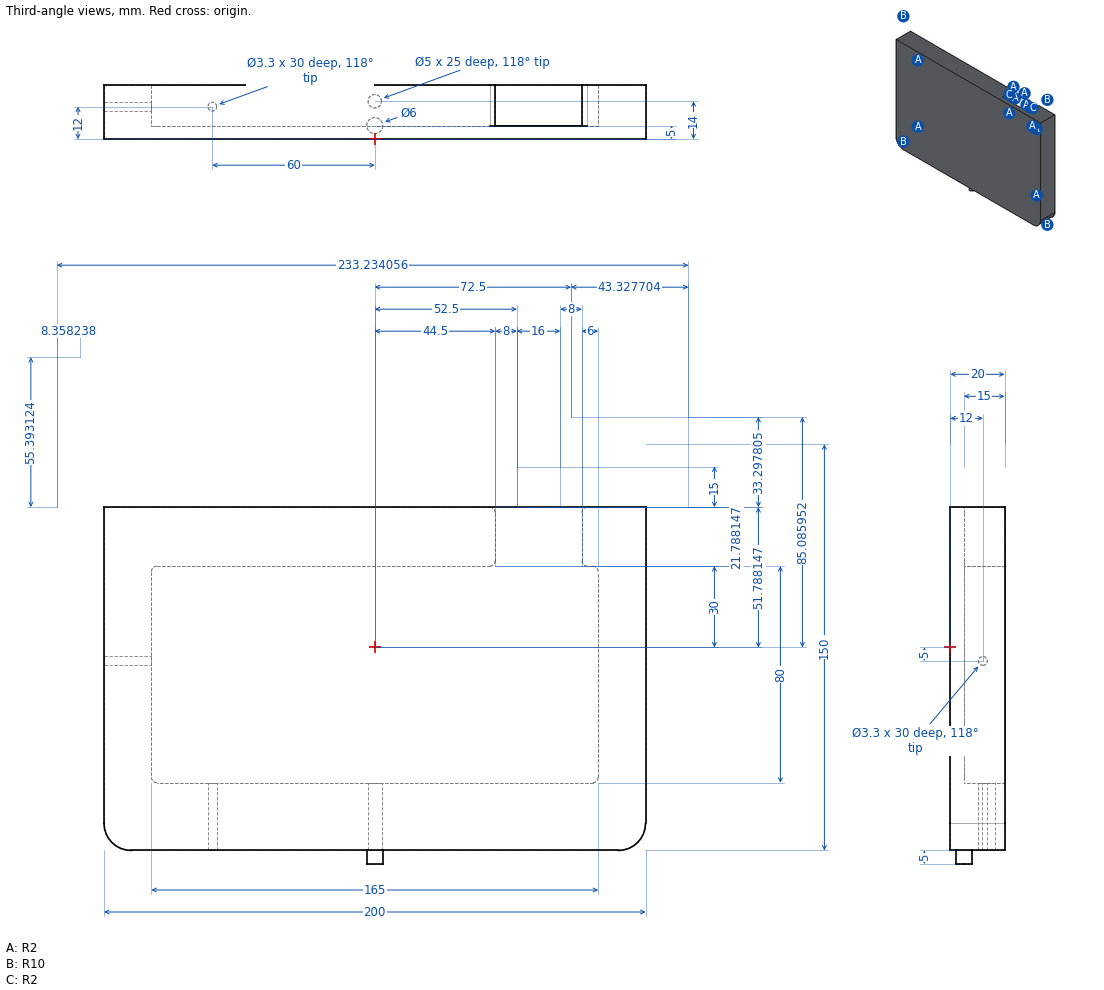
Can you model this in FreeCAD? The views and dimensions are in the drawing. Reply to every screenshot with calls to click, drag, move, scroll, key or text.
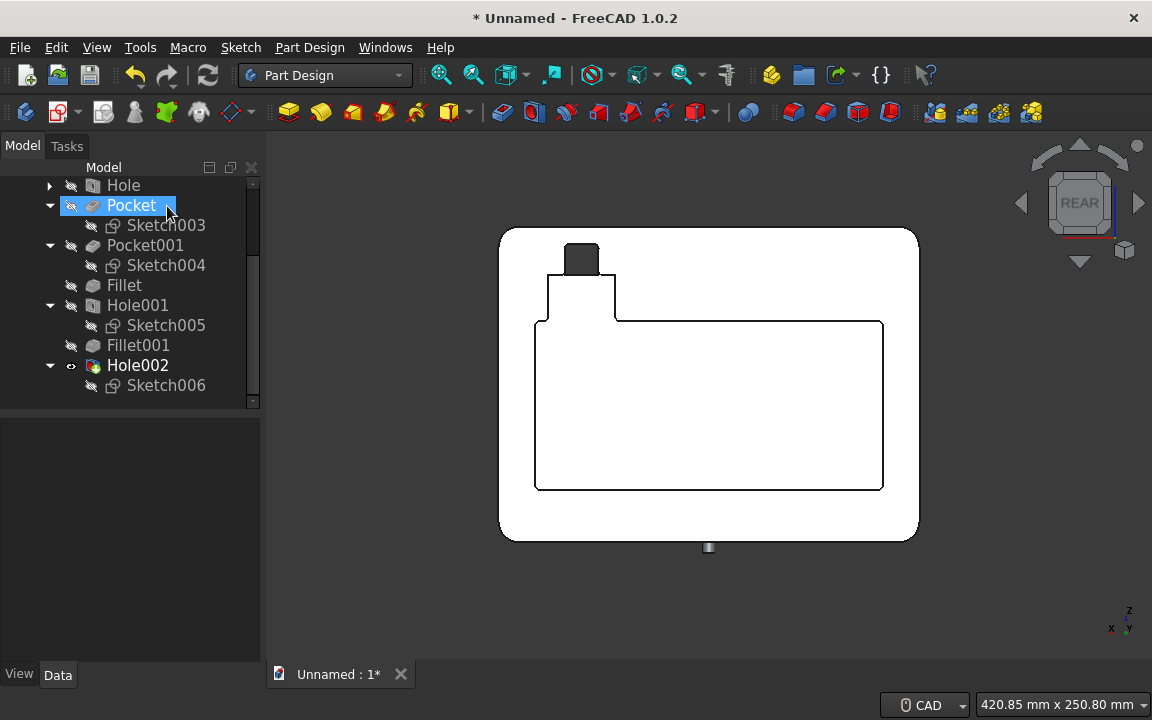
click(889, 293)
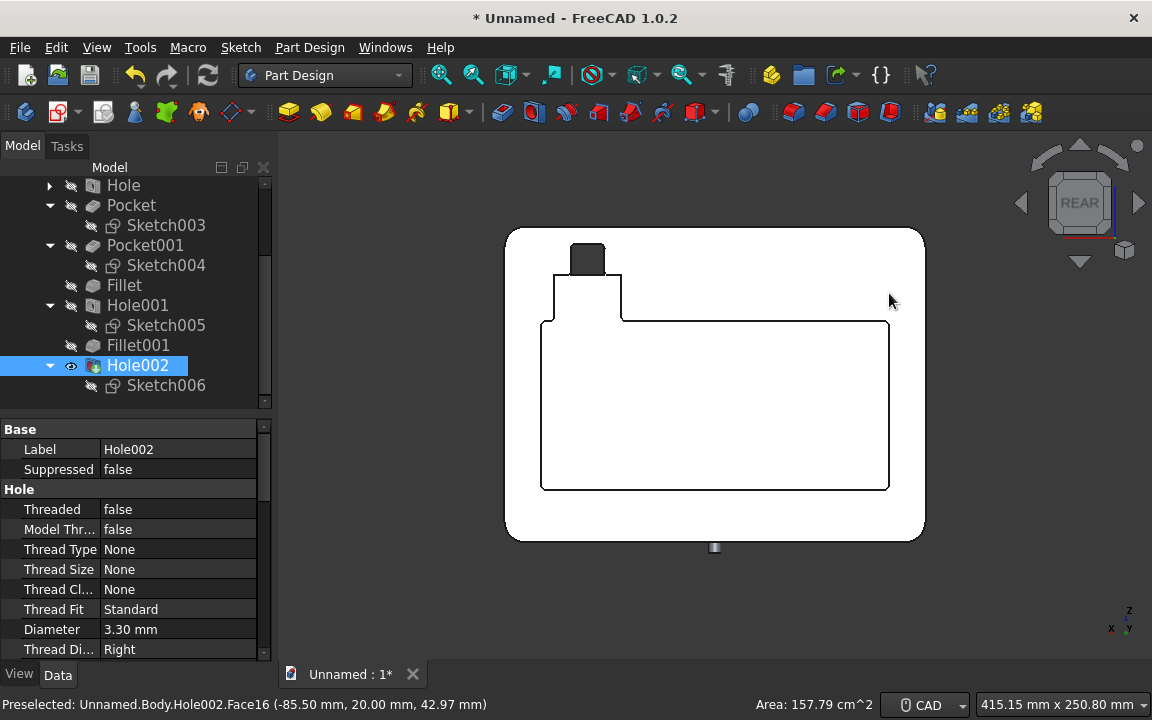
click(58, 112)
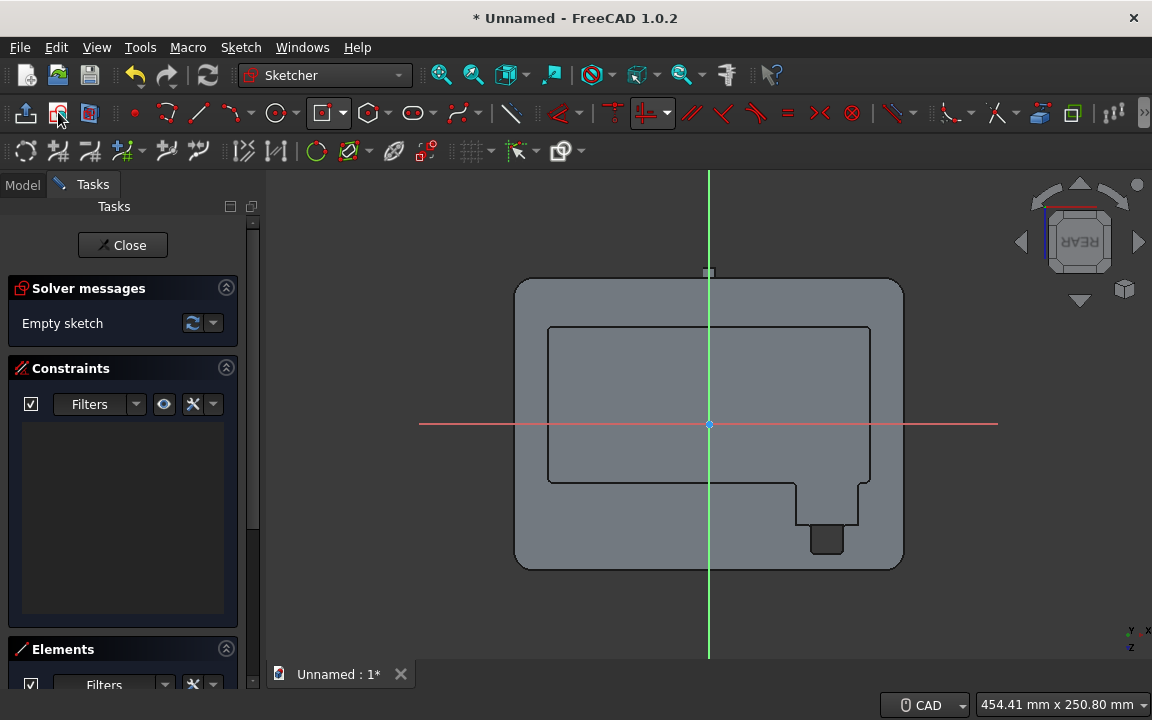
scroll(338, 198, down, 1)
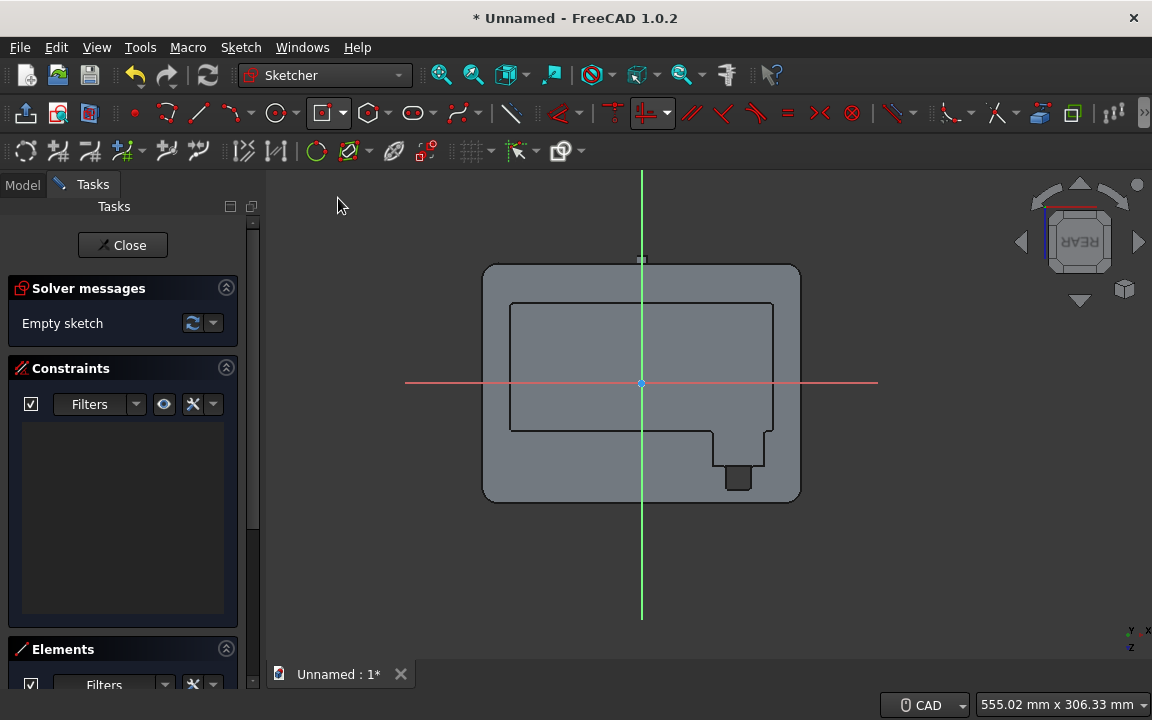
key(g)
key(m)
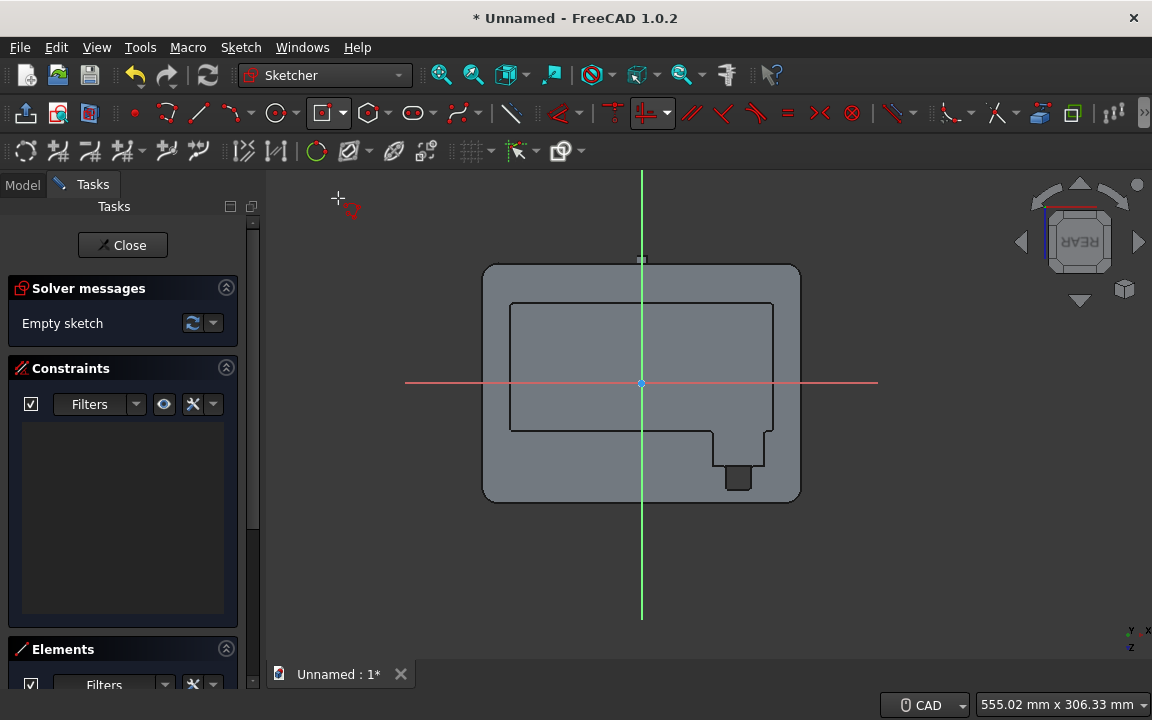
click(757, 519)
click(827, 519)
click(827, 466)
click(454, 466)
click(468, 554)
click(757, 520)
key(Escape)
key(Escape)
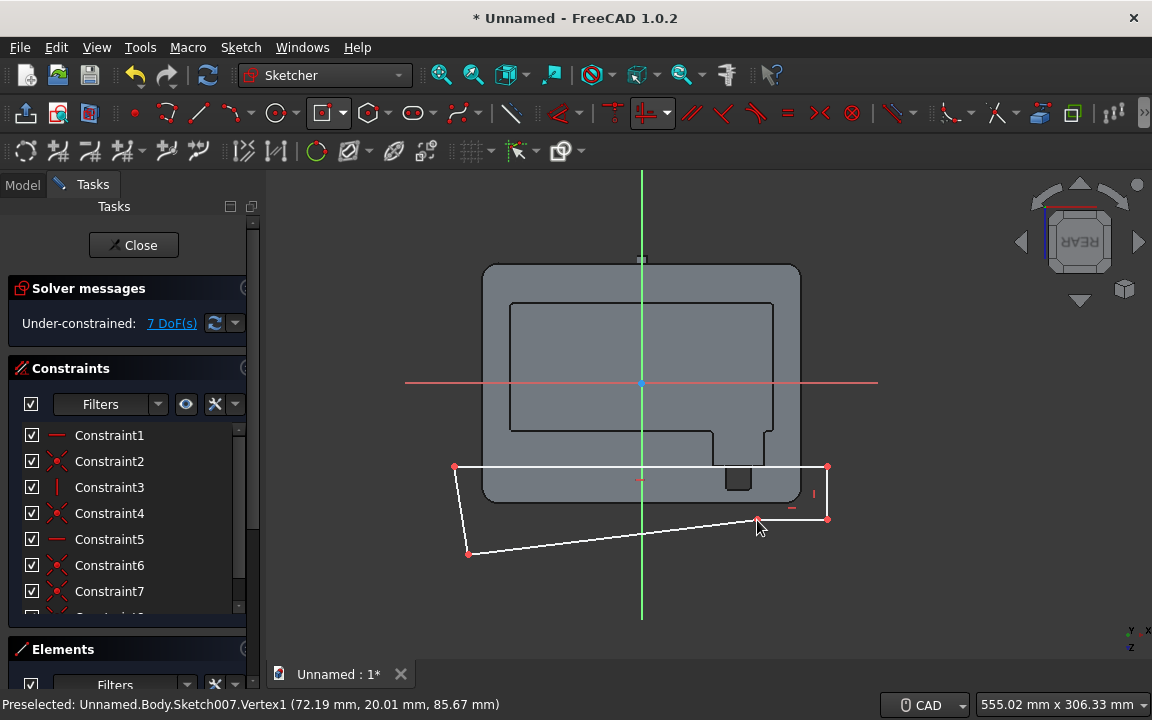
click(558, 114)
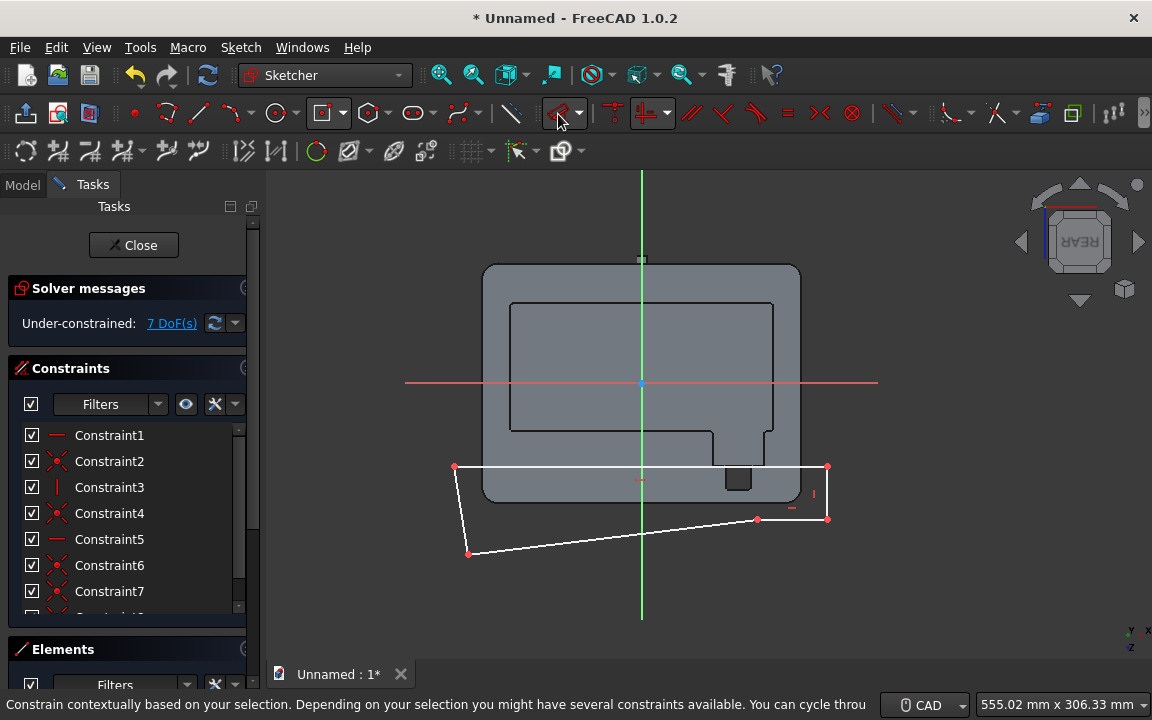
click(757, 520)
click(699, 349)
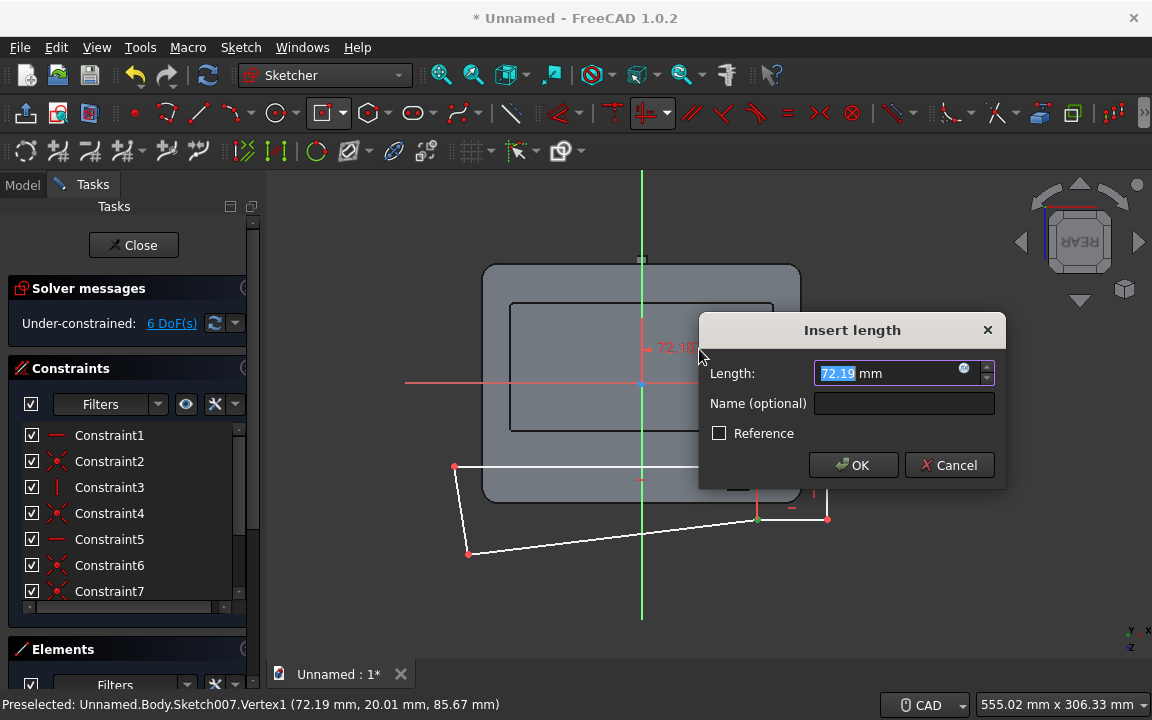
text(72.5)
key(Return)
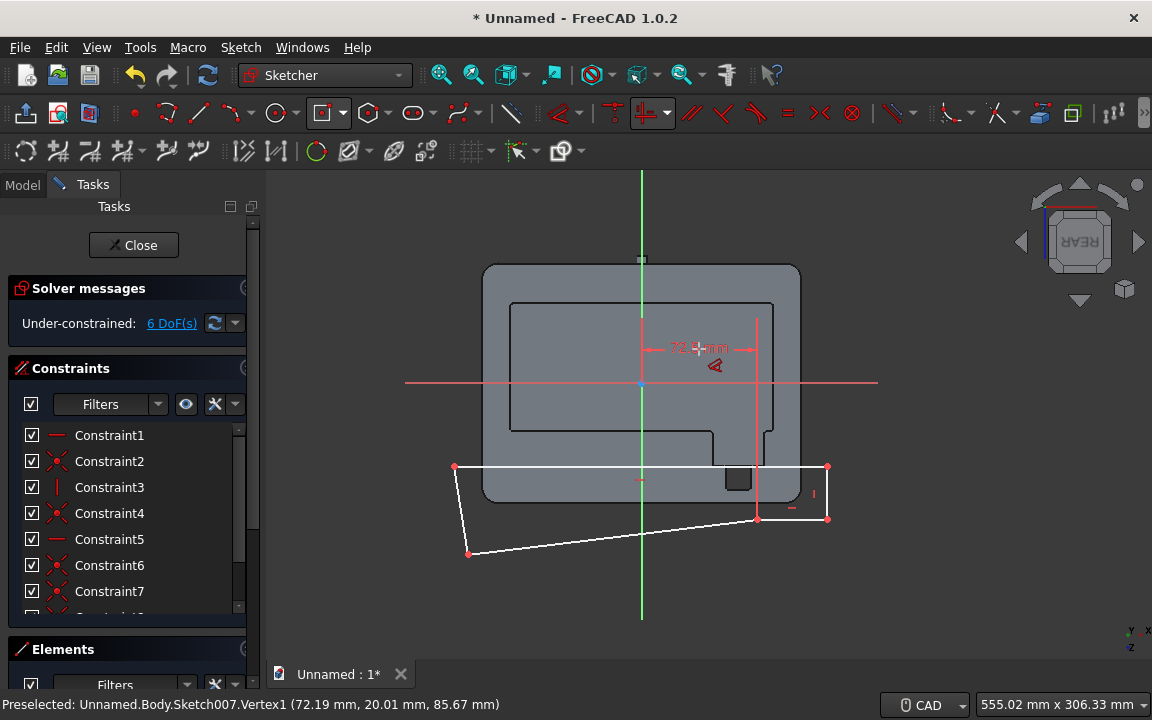
click(778, 520)
click(792, 554)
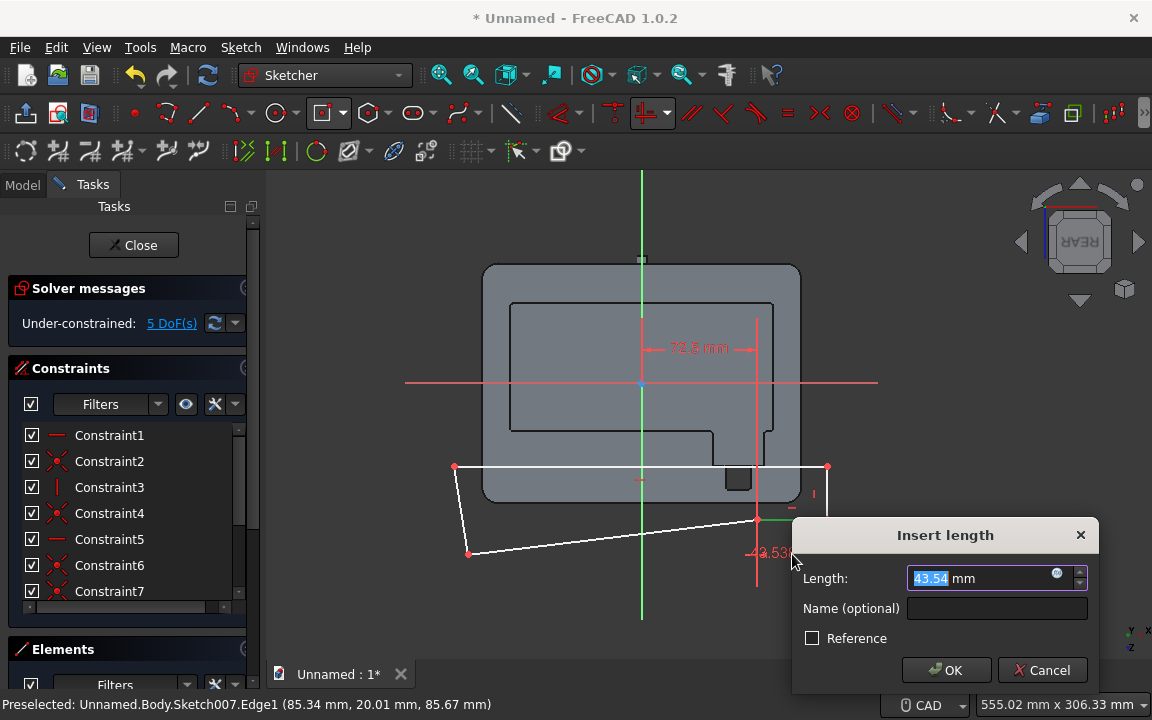
text(43.327704)
key(Return)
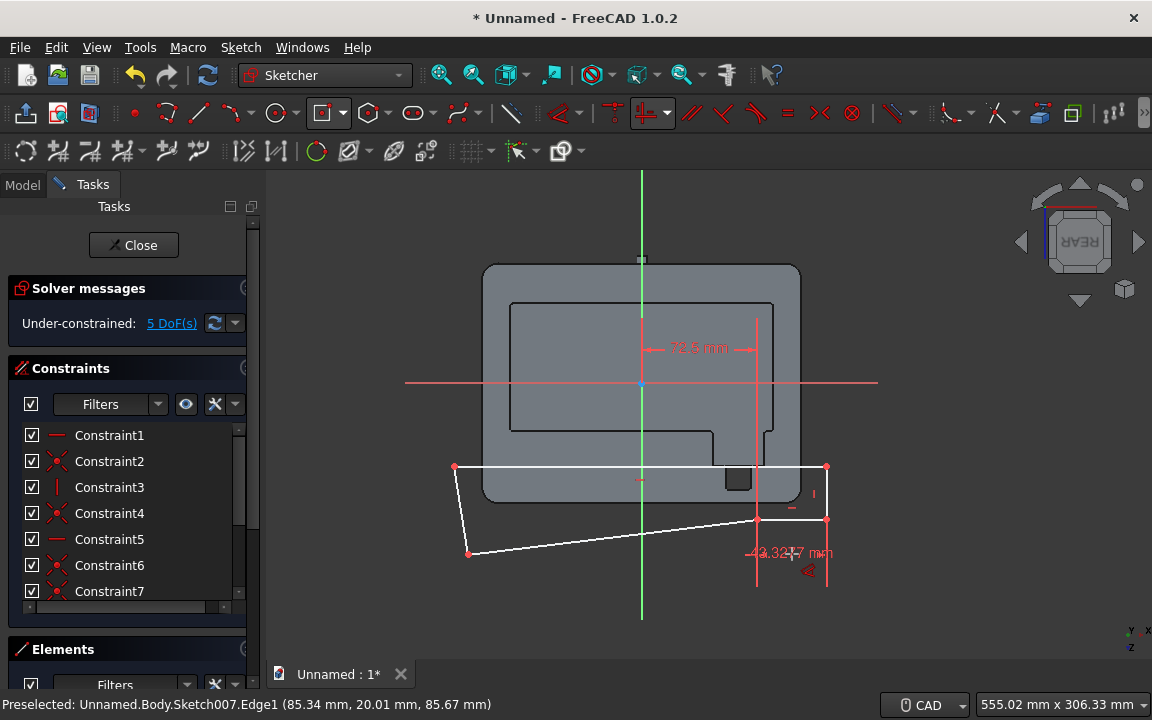
click(827, 504)
click(861, 494)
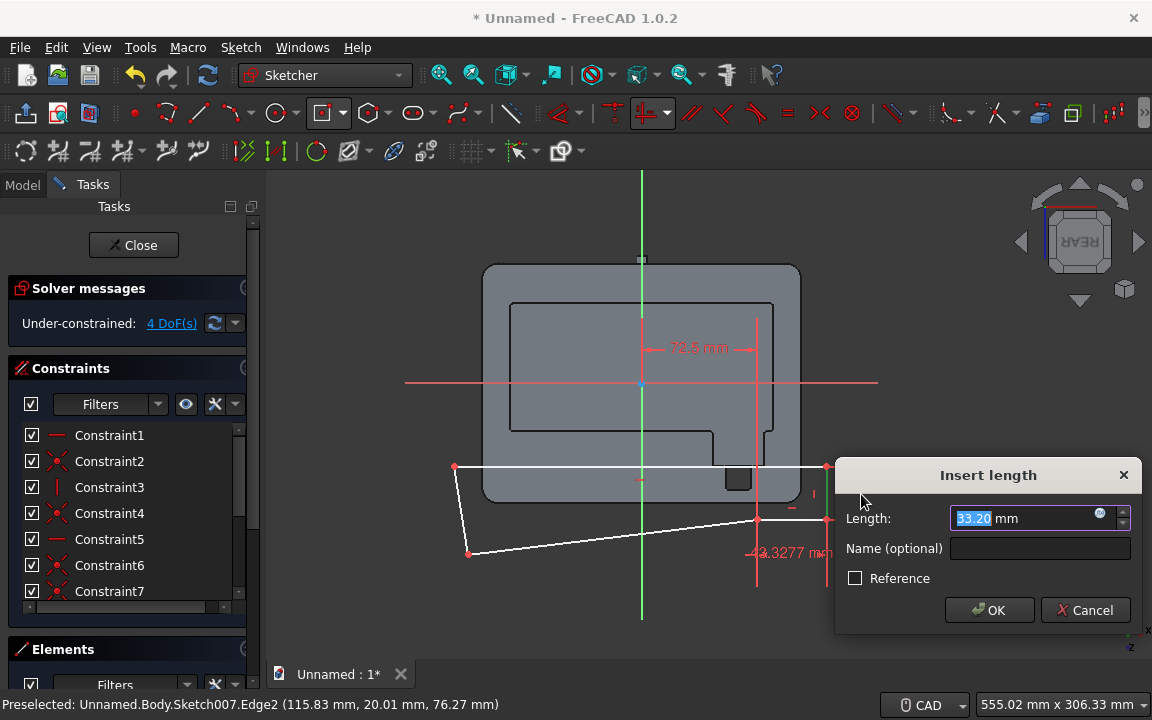
text(33.297805)
key(Return)